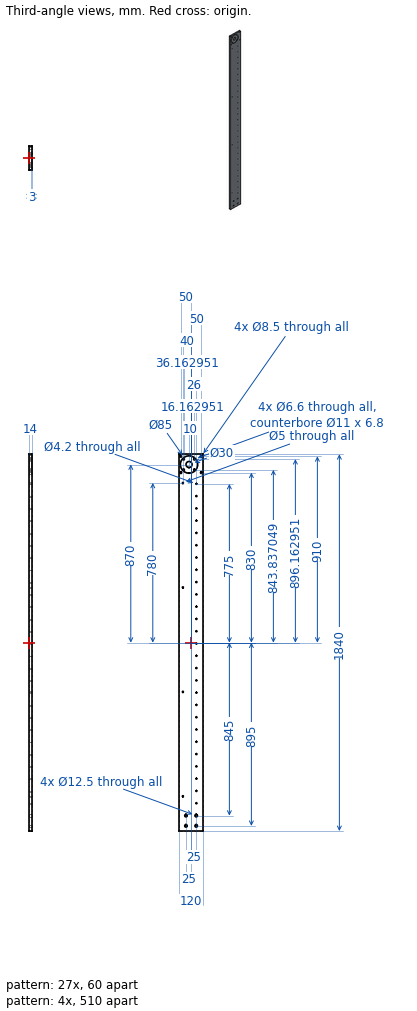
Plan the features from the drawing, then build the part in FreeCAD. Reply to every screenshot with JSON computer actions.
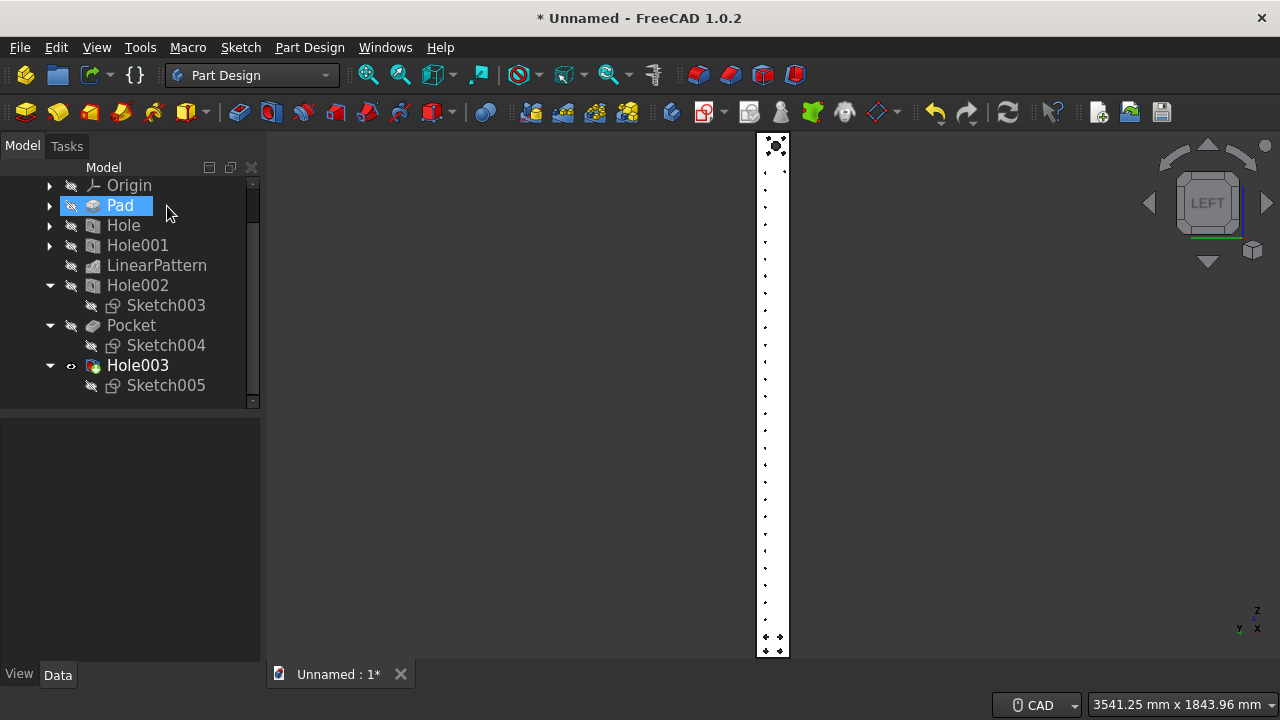
{"action": "left_click", "coordinate": [116, 366]}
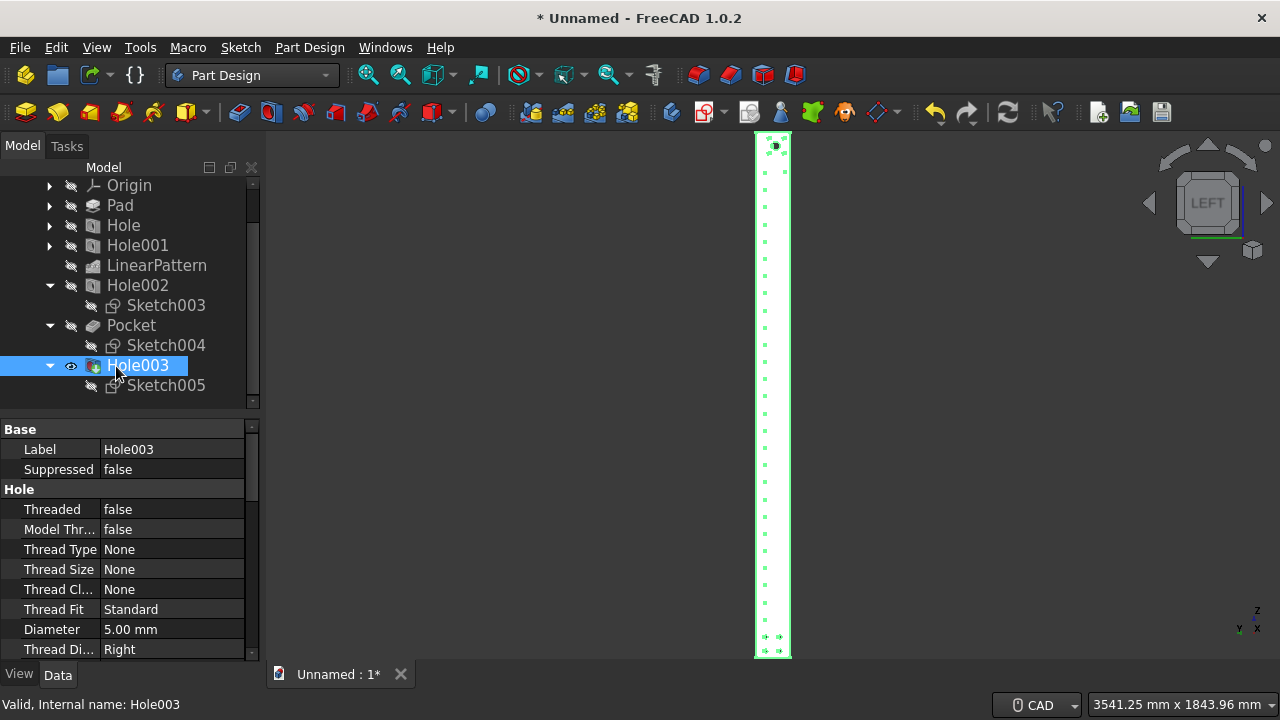
{"action": "left_click", "coordinate": [564, 112]}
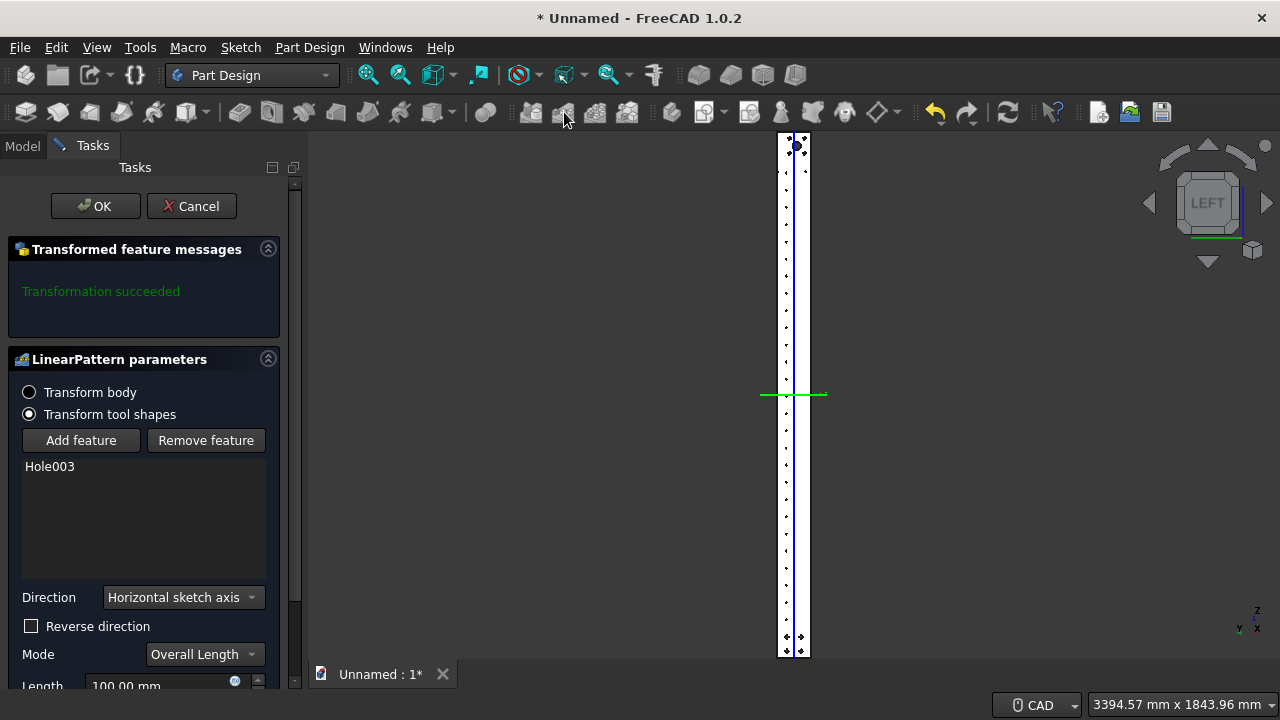
{"action": "left_click", "coordinate": [184, 598]}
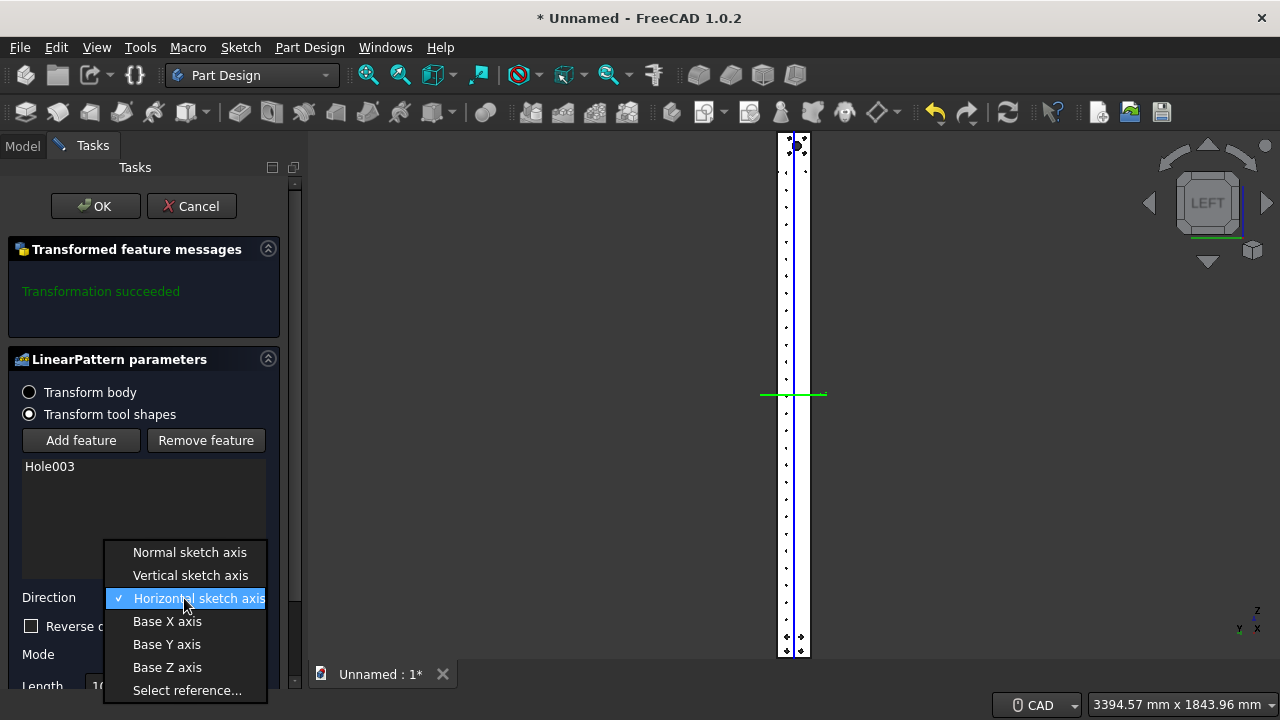
{"action": "left_click", "coordinate": [184, 668]}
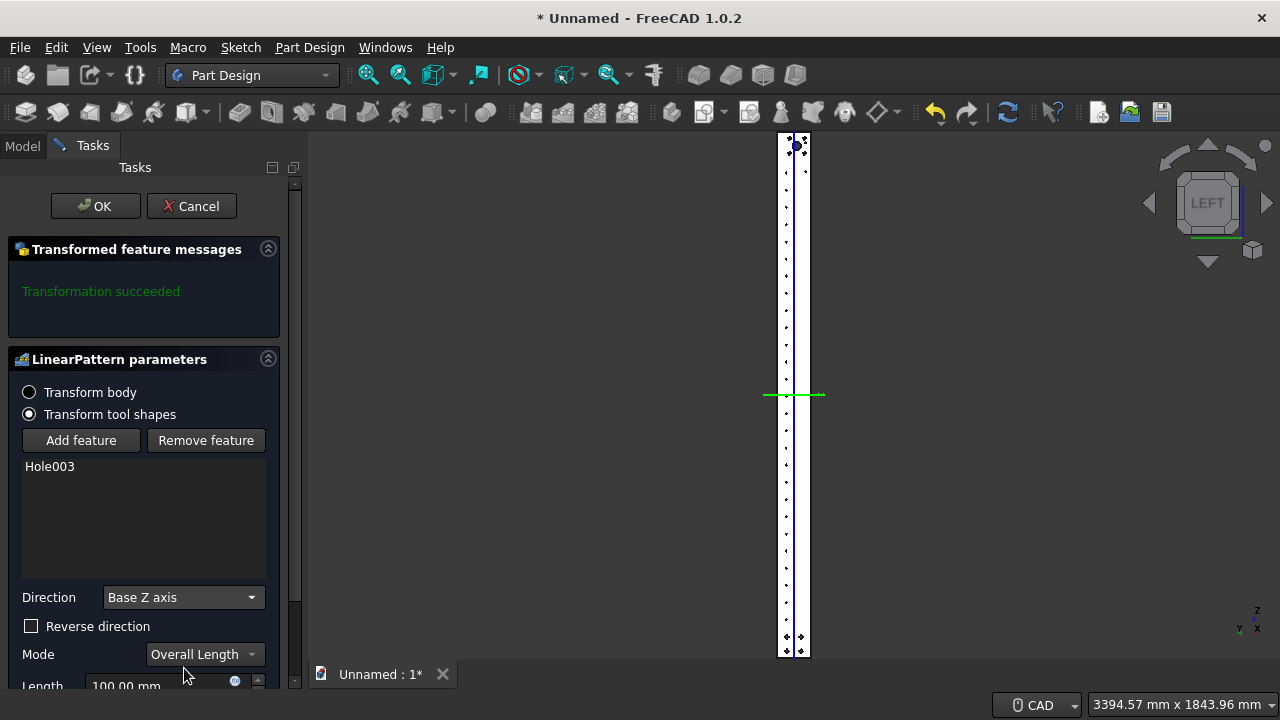
{"action": "left_click", "coordinate": [206, 654]}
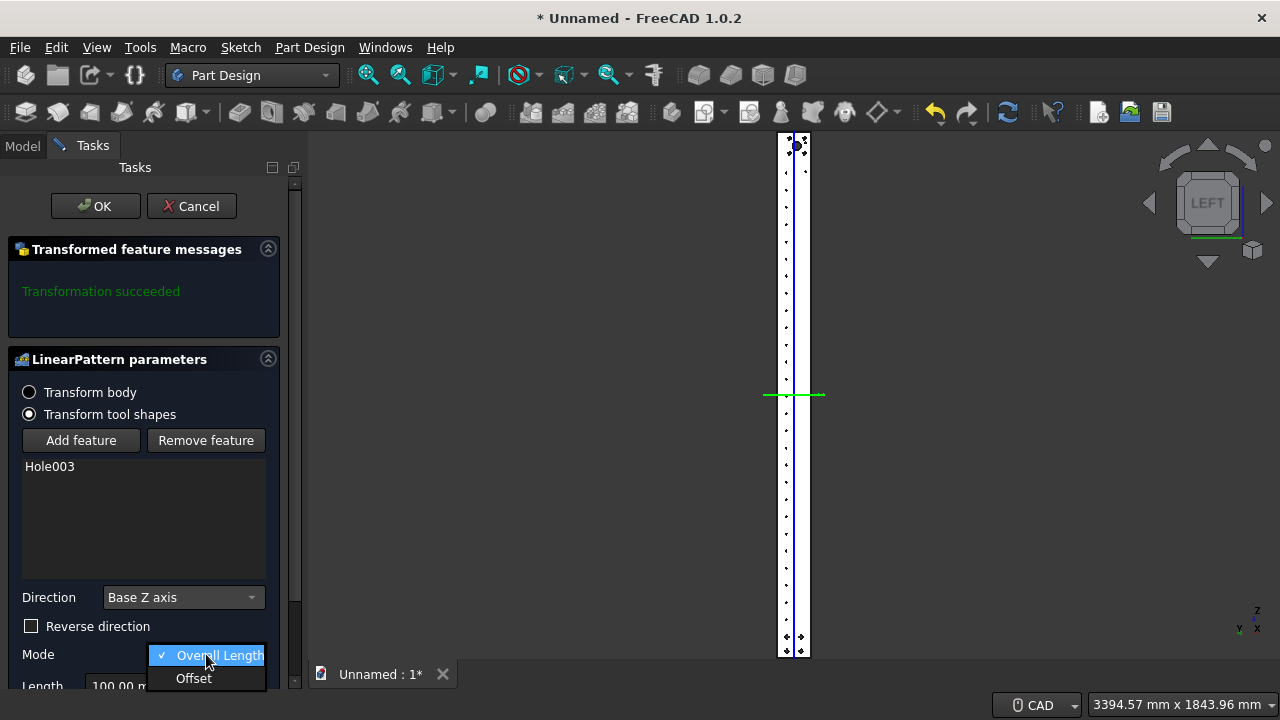
{"action": "left_click", "coordinate": [206, 678]}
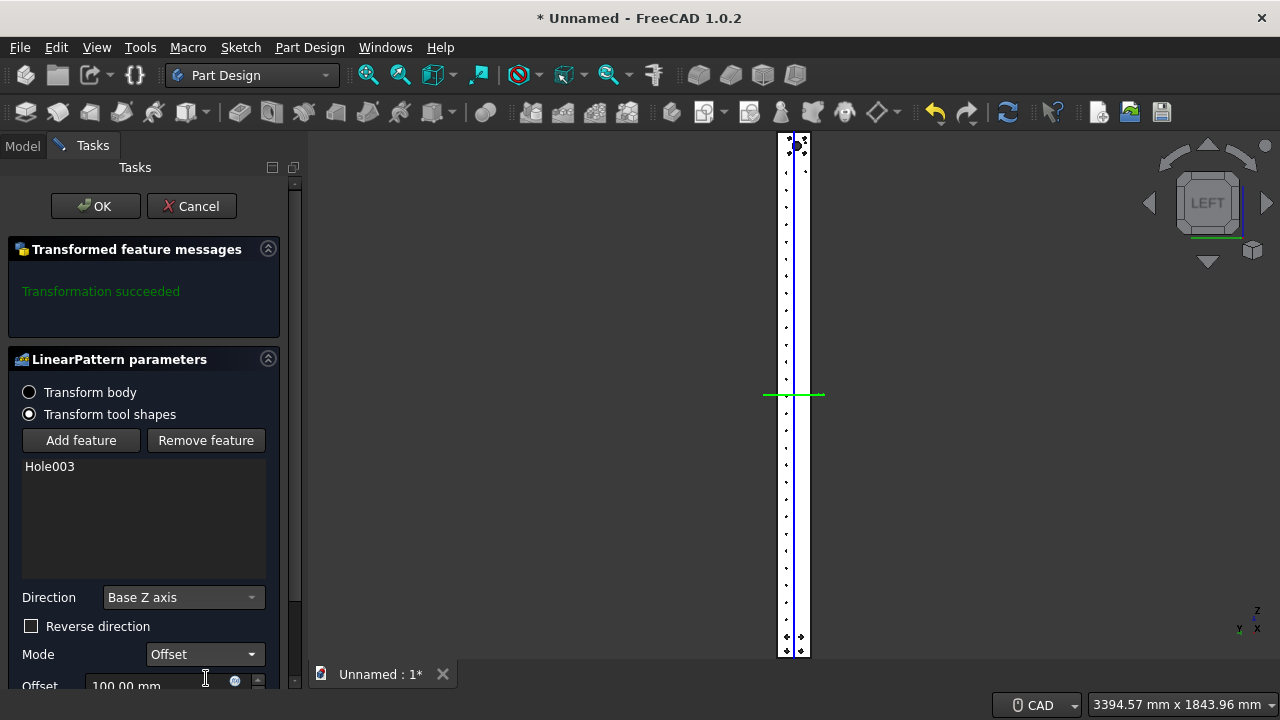
{"action": "scroll", "coordinate": [295, 432], "scroll_direction": "down", "scroll_amount": 2}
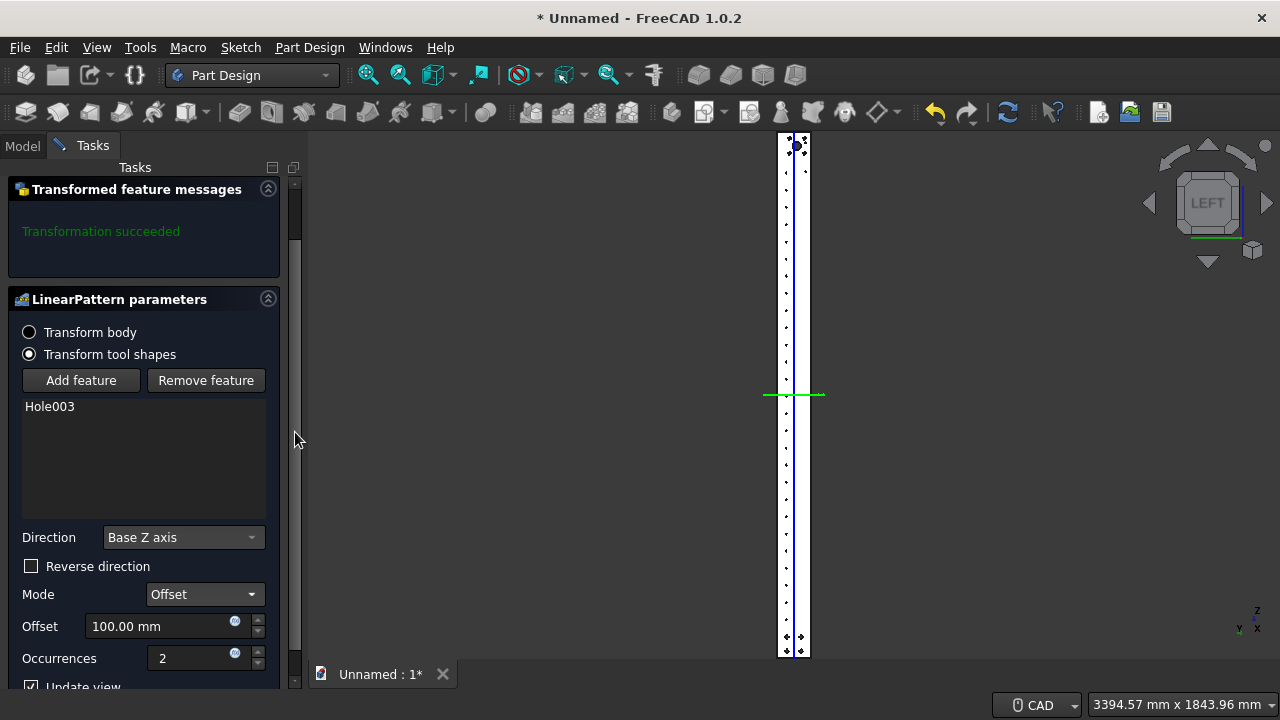
{"action": "triple_click", "coordinate": [168, 596]}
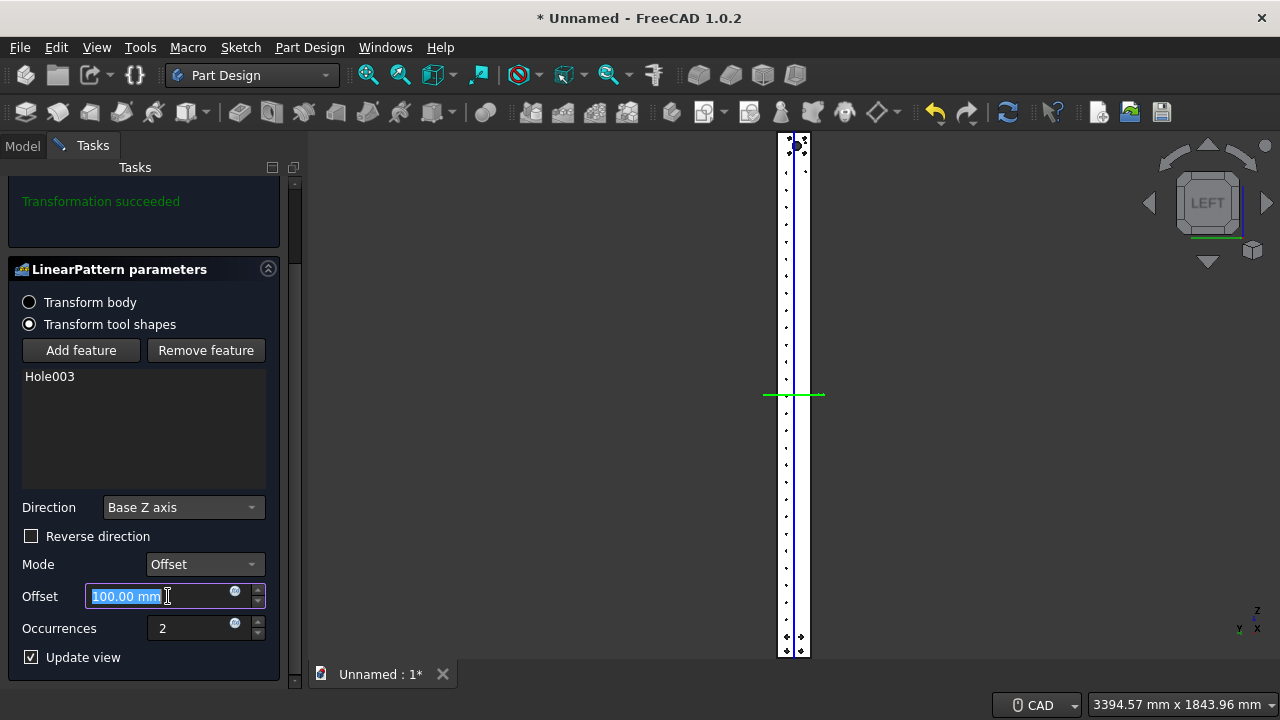
{"action": "type", "text": "510"}
{"action": "key", "text": "Tab"}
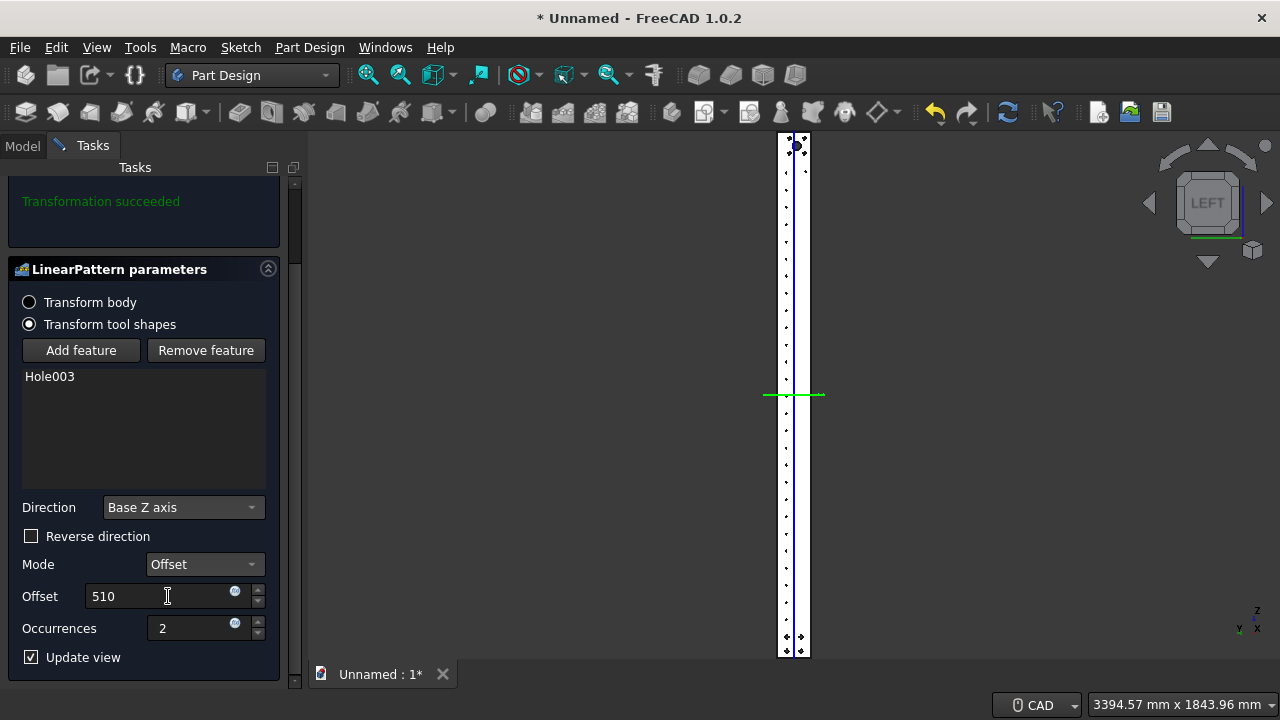
{"action": "triple_click", "coordinate": [198, 628]}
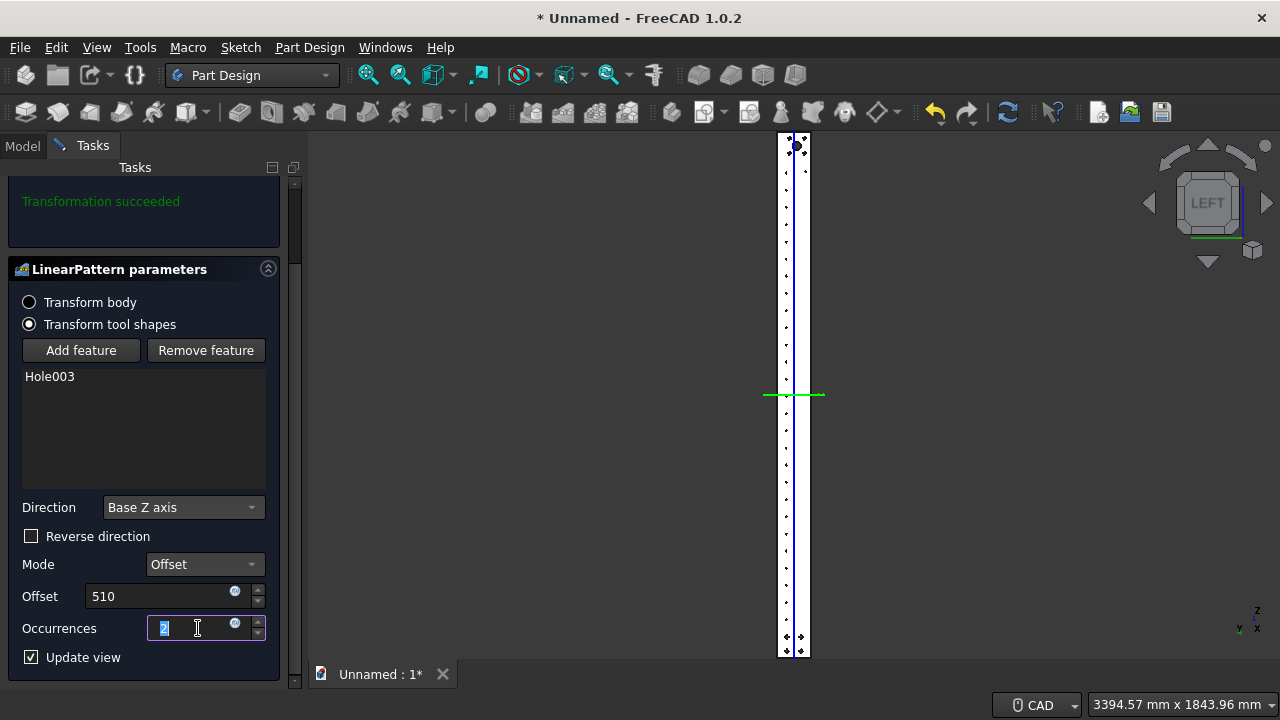
{"action": "type", "text": "4"}
{"action": "key", "text": "Tab"}